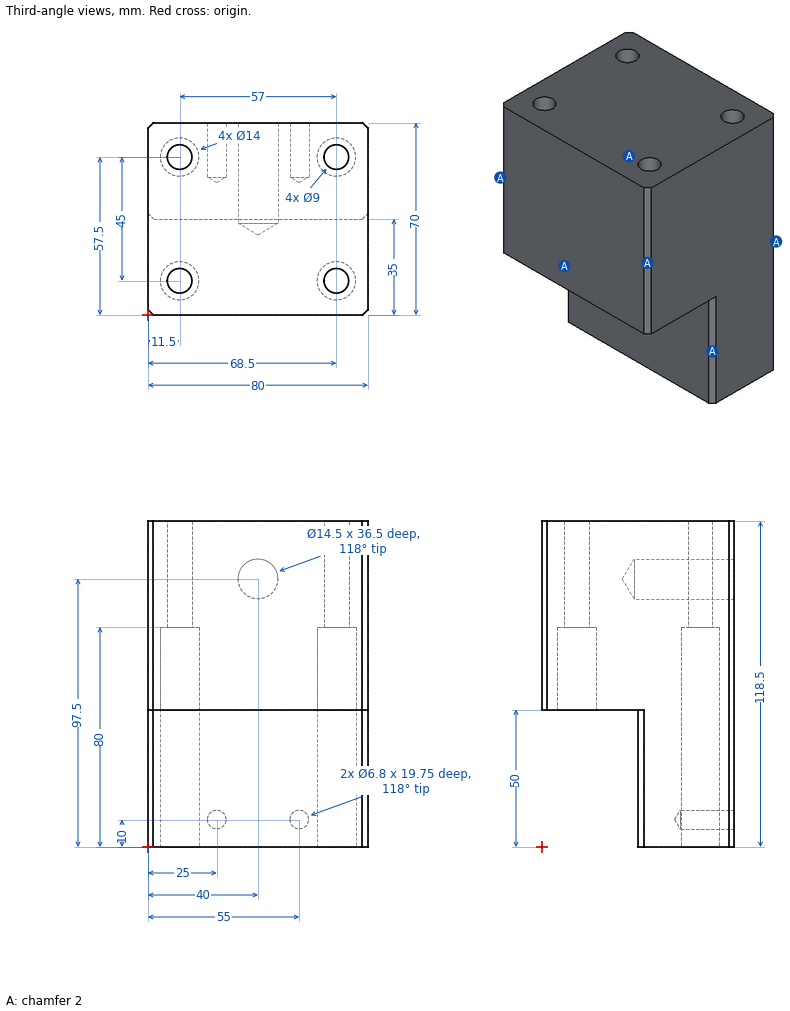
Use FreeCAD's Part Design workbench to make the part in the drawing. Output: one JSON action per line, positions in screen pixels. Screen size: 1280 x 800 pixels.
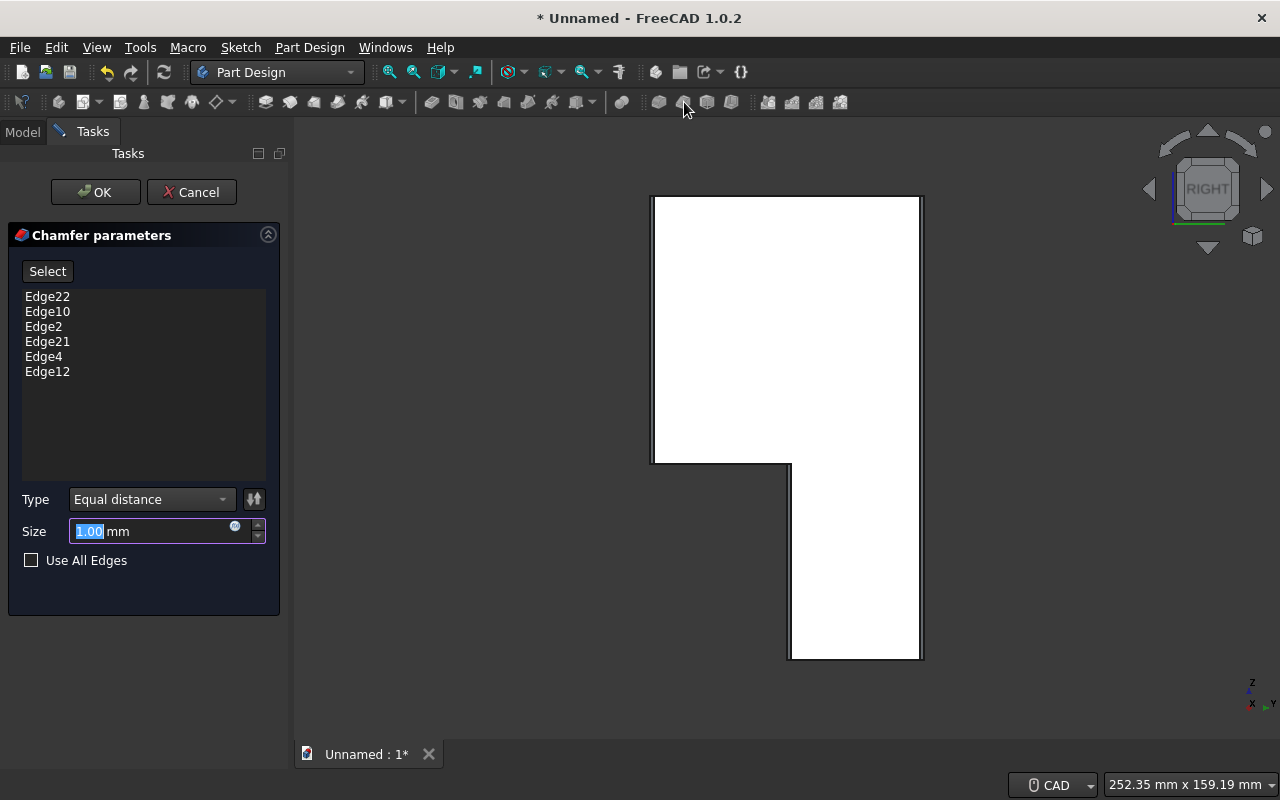
{"action": "type", "text": "2"}
{"action": "key", "text": "Tab"}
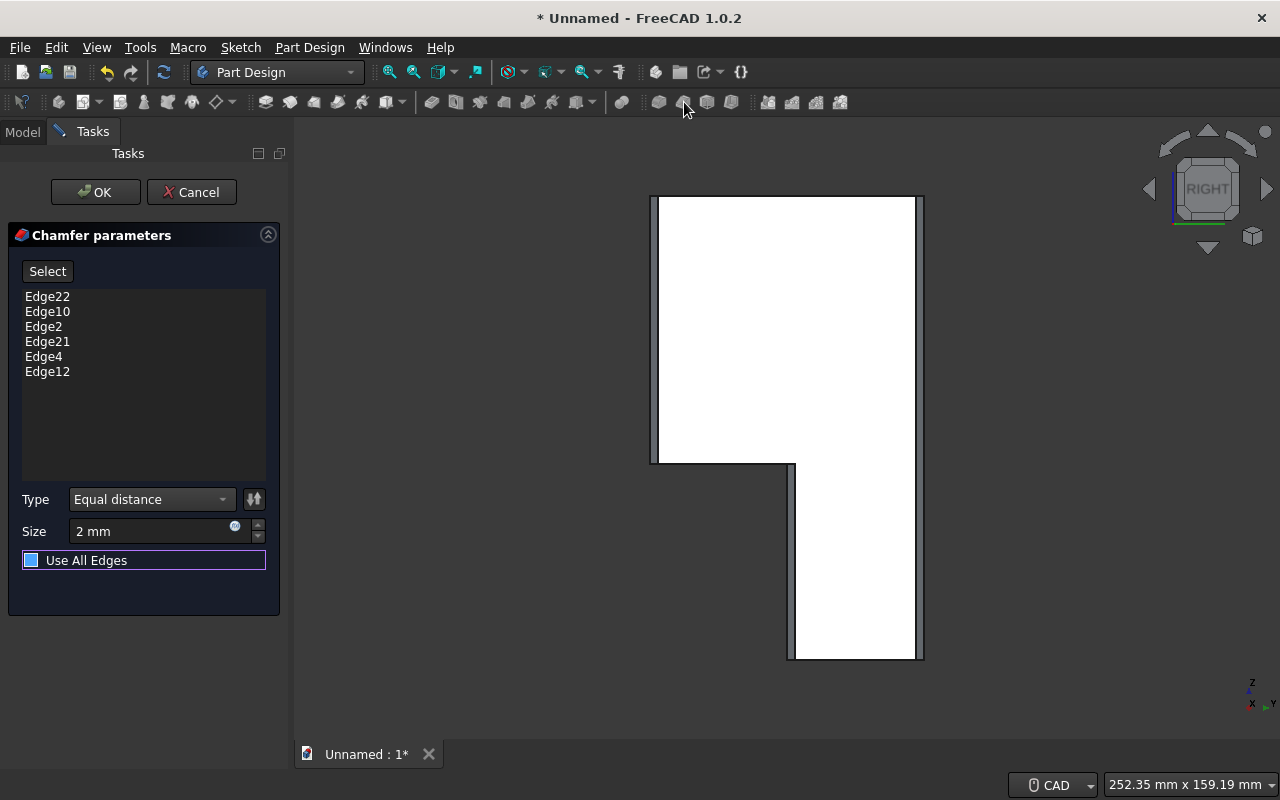
{"action": "left_click", "coordinate": [96, 192]}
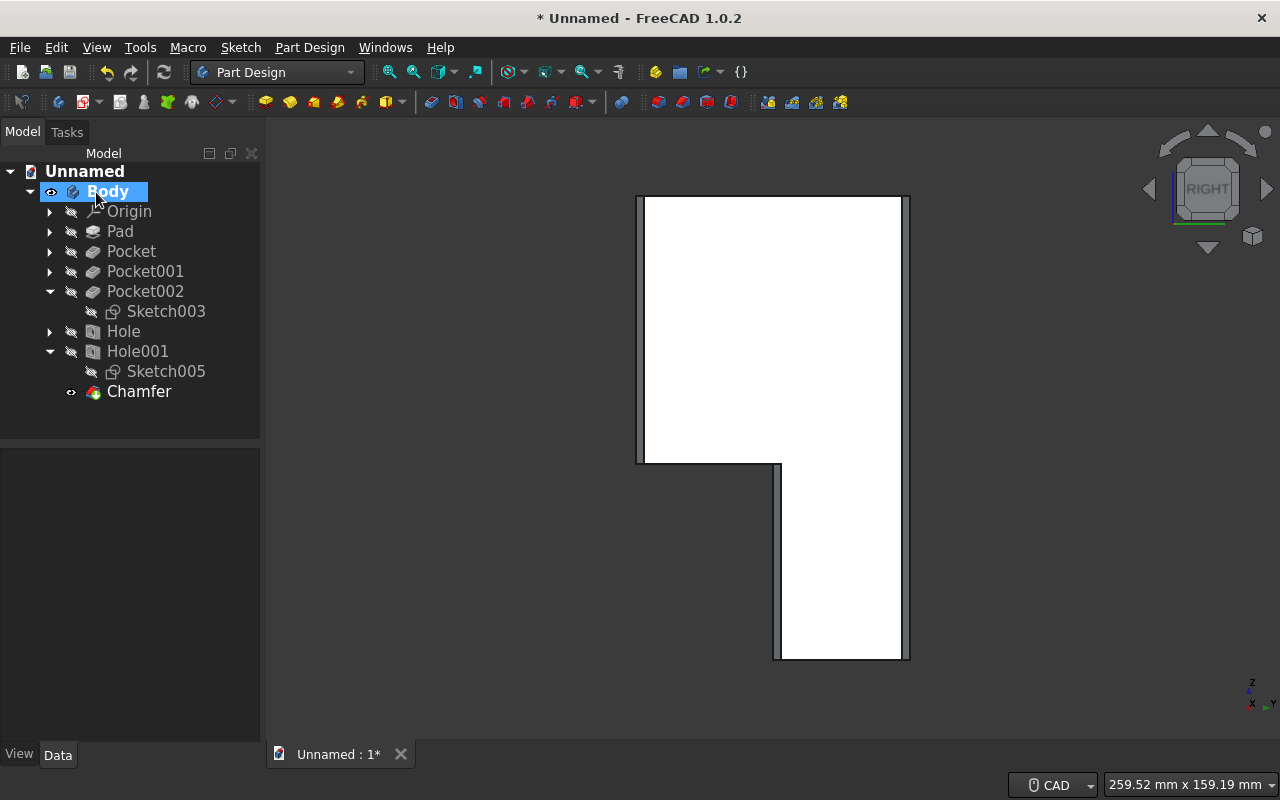
{"action": "key", "text": "0"}